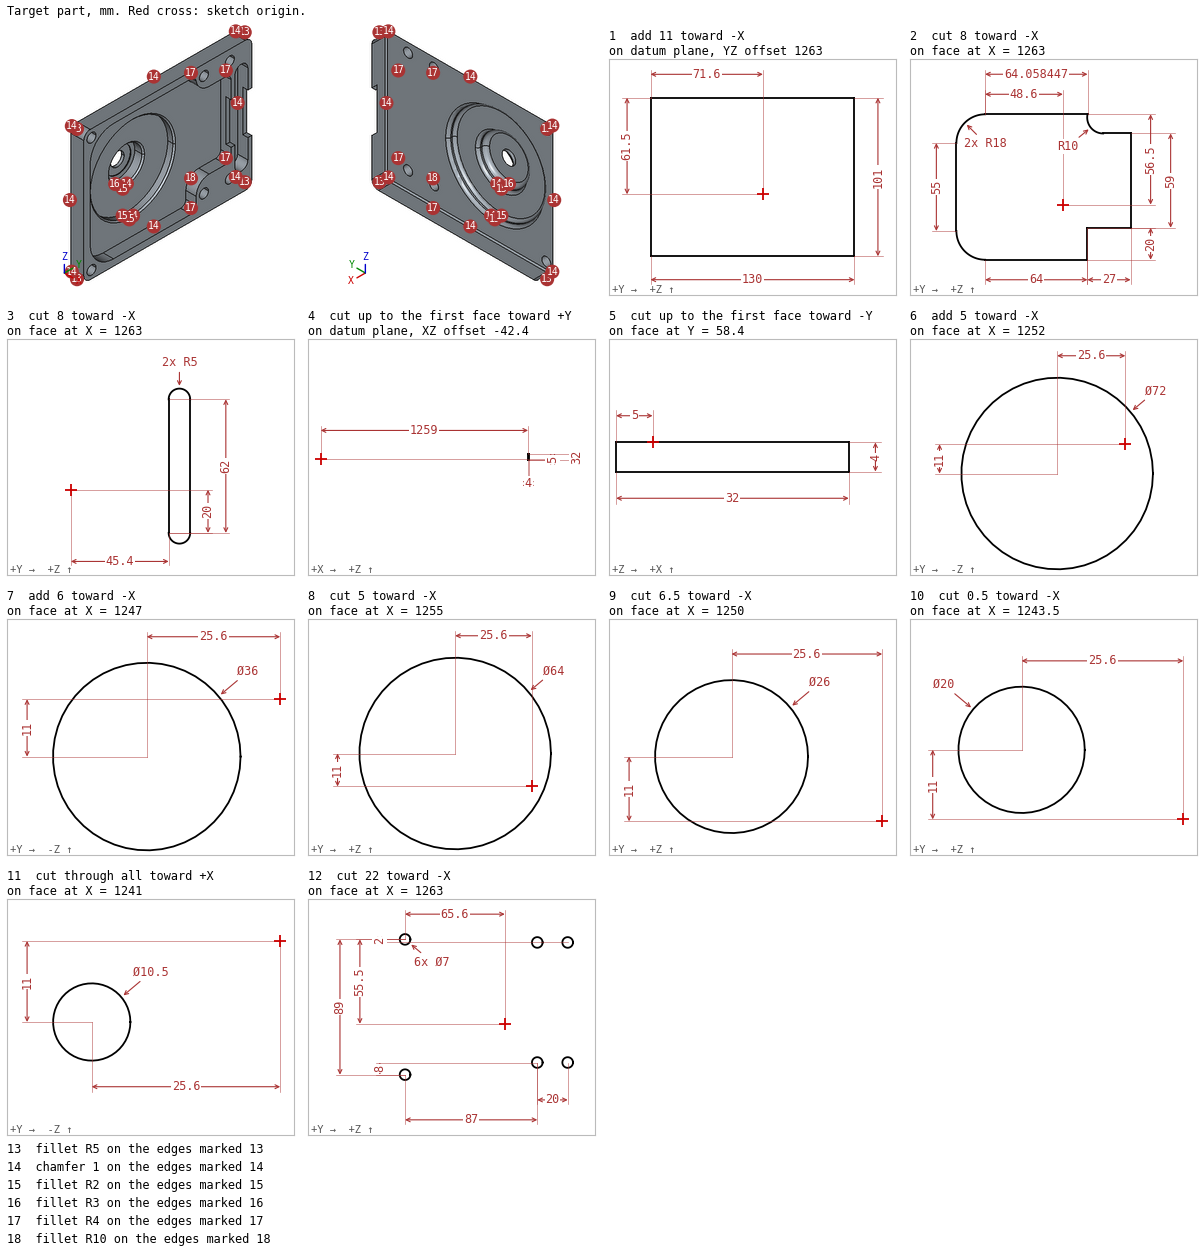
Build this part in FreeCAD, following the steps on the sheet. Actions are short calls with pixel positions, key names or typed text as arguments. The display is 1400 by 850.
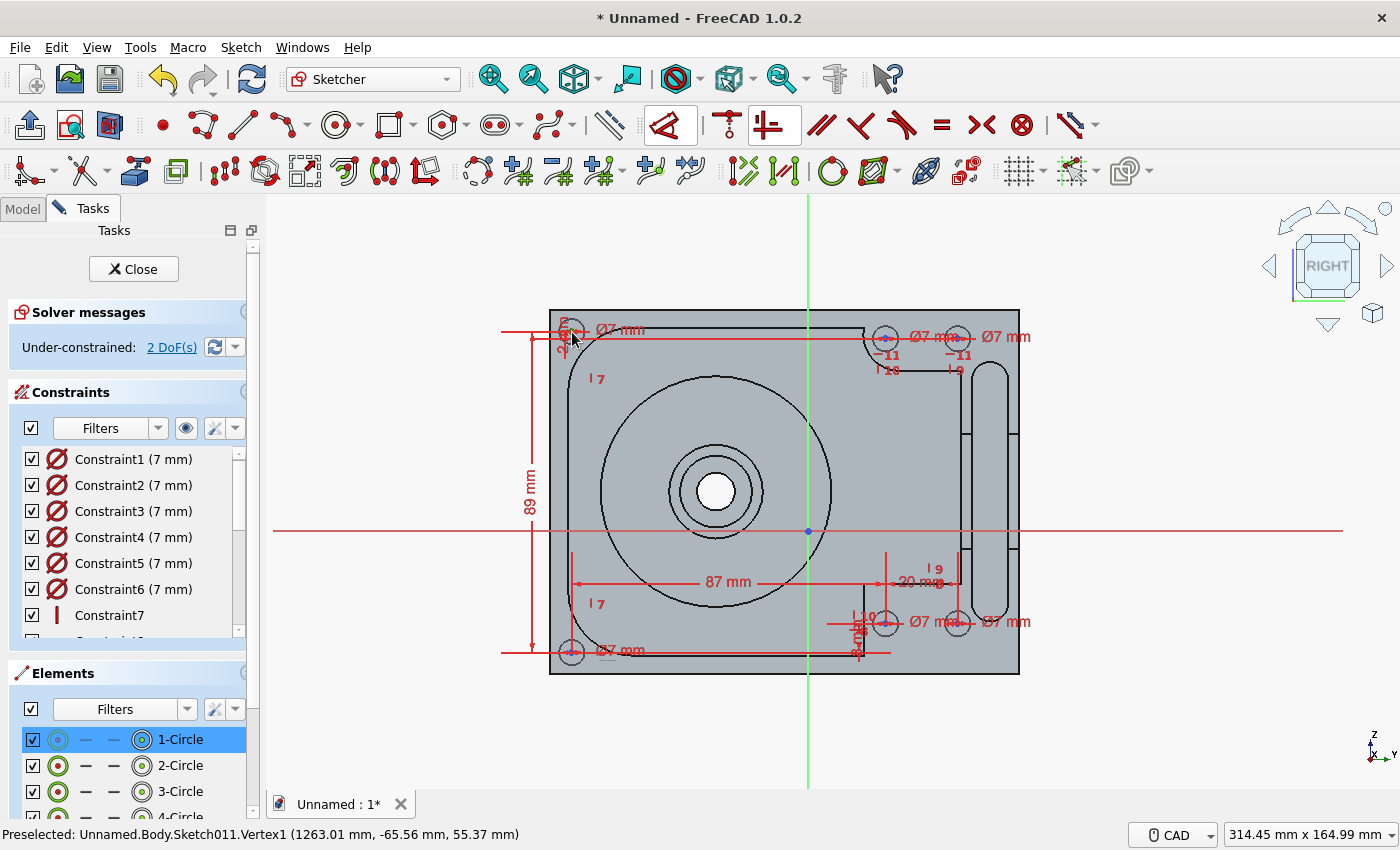
click(692, 126)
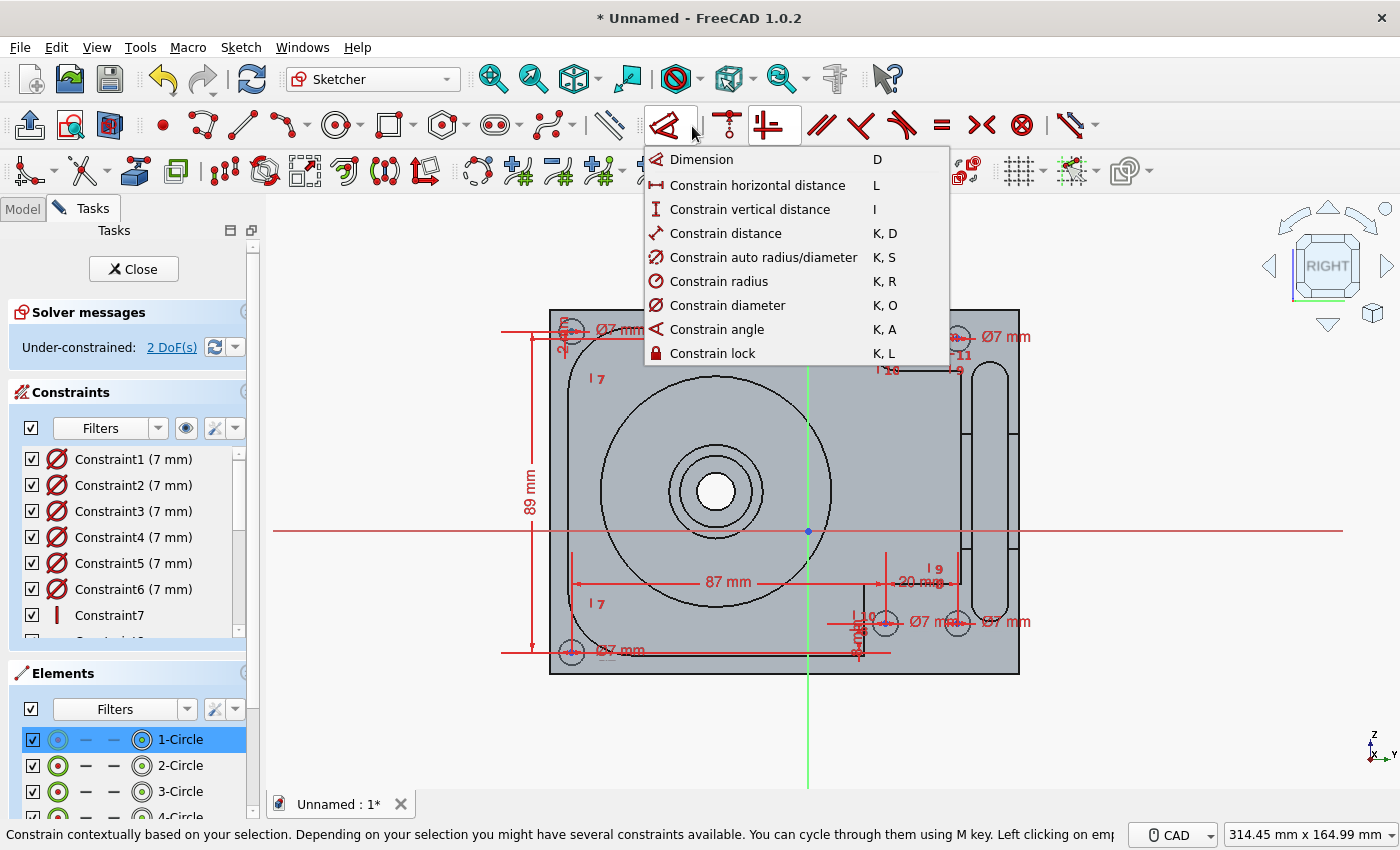
click(797, 185)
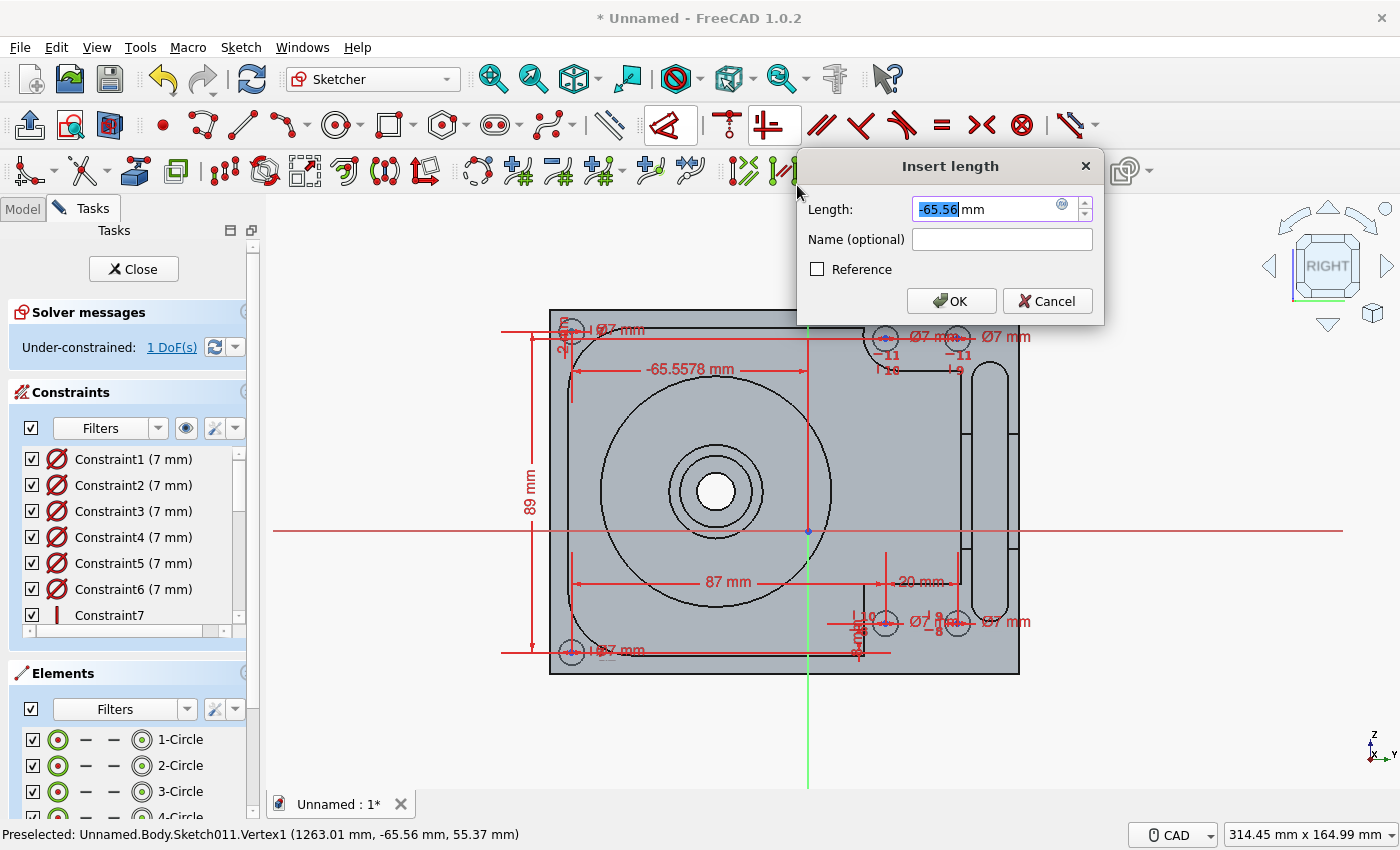
text(-65.6)
key(Return)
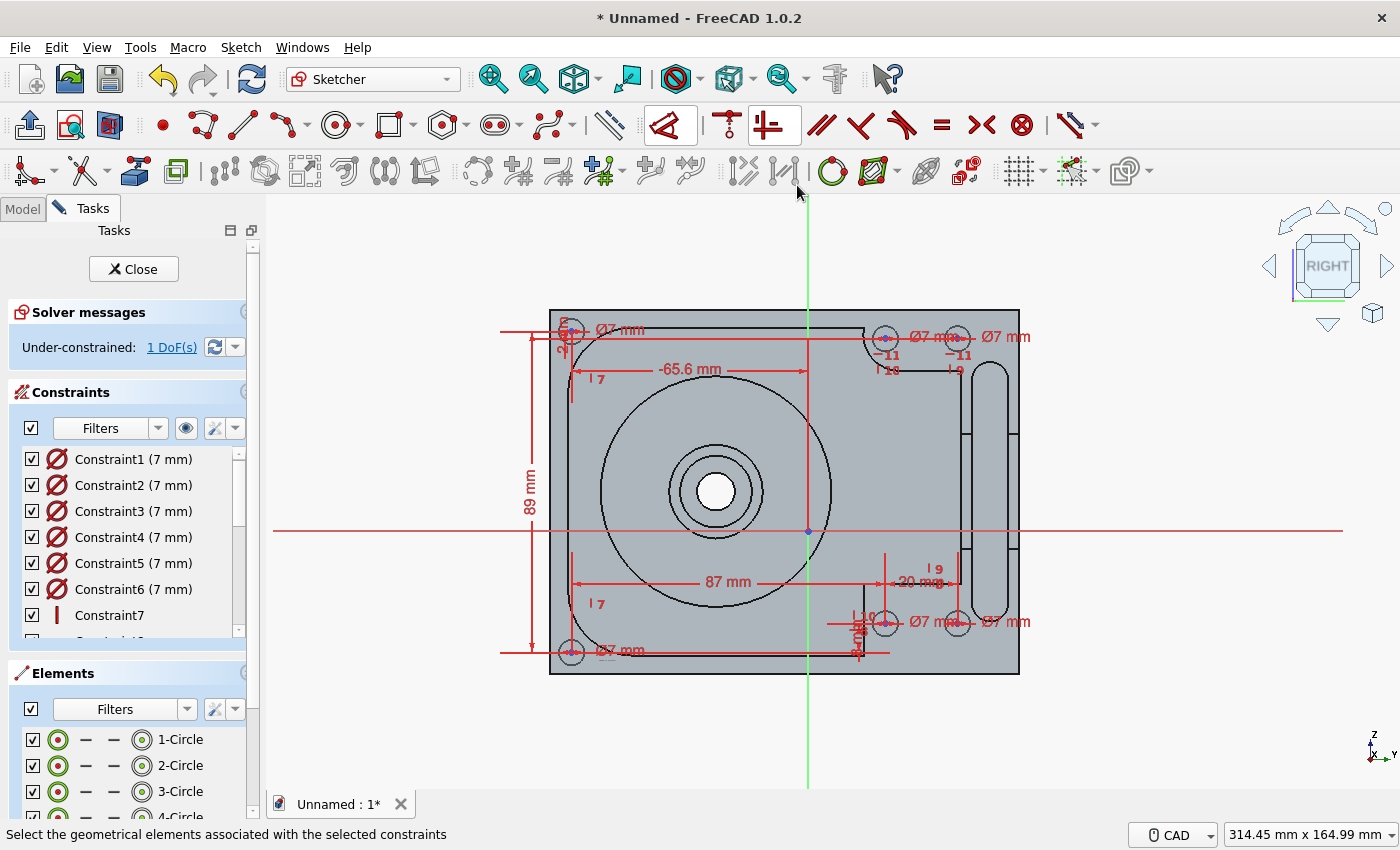
click(572, 332)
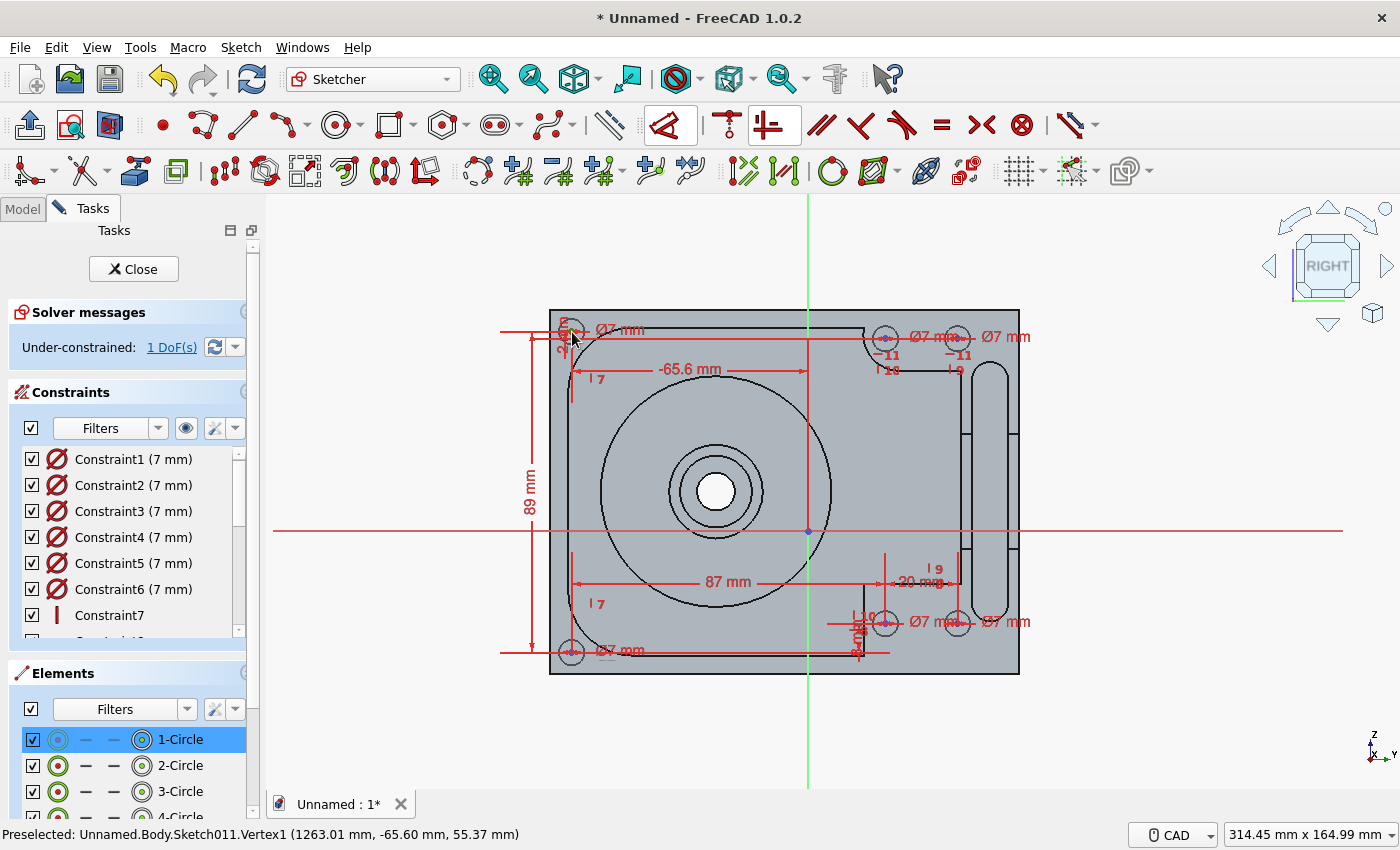
key(i)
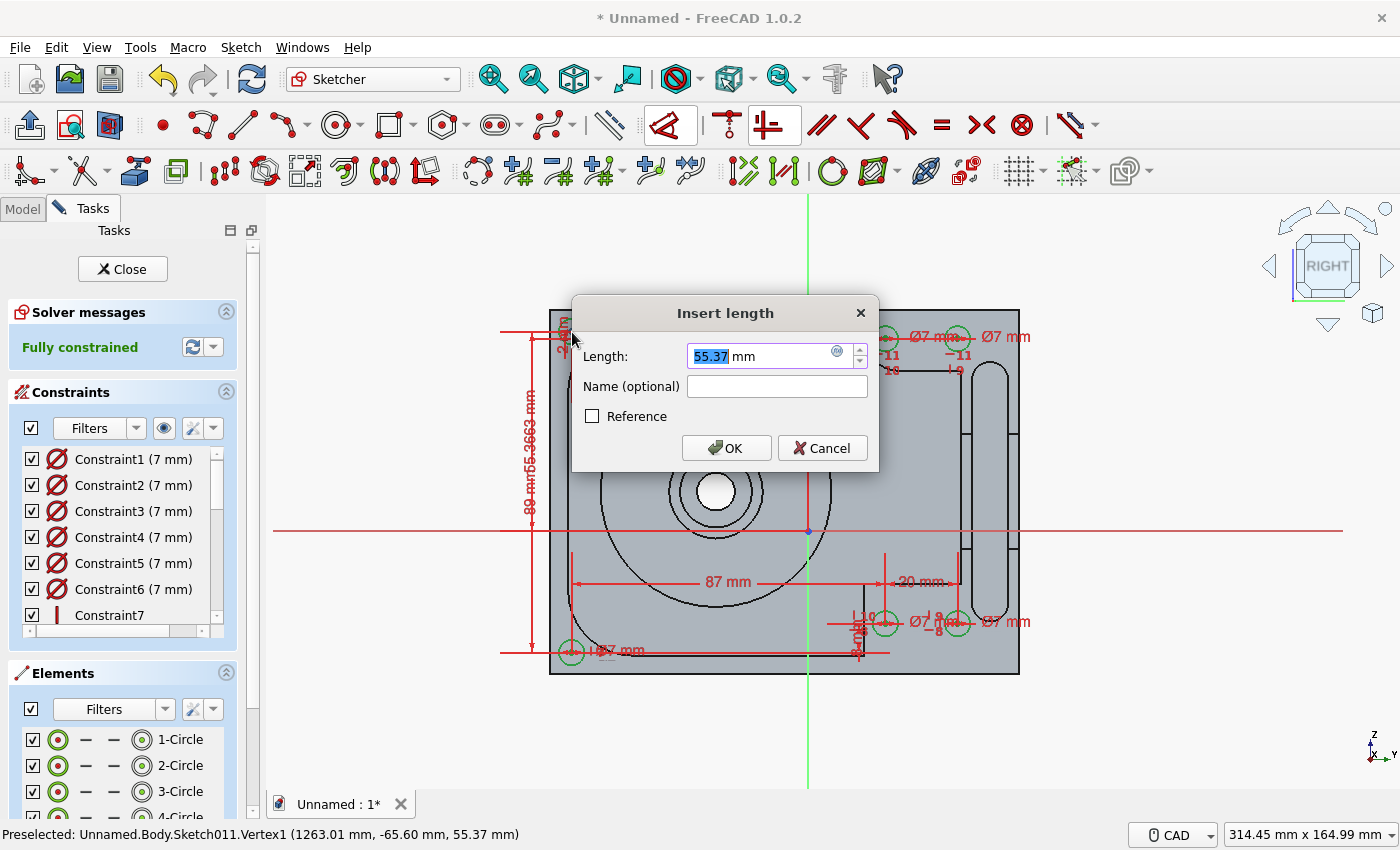
text(55.5)
key(Return)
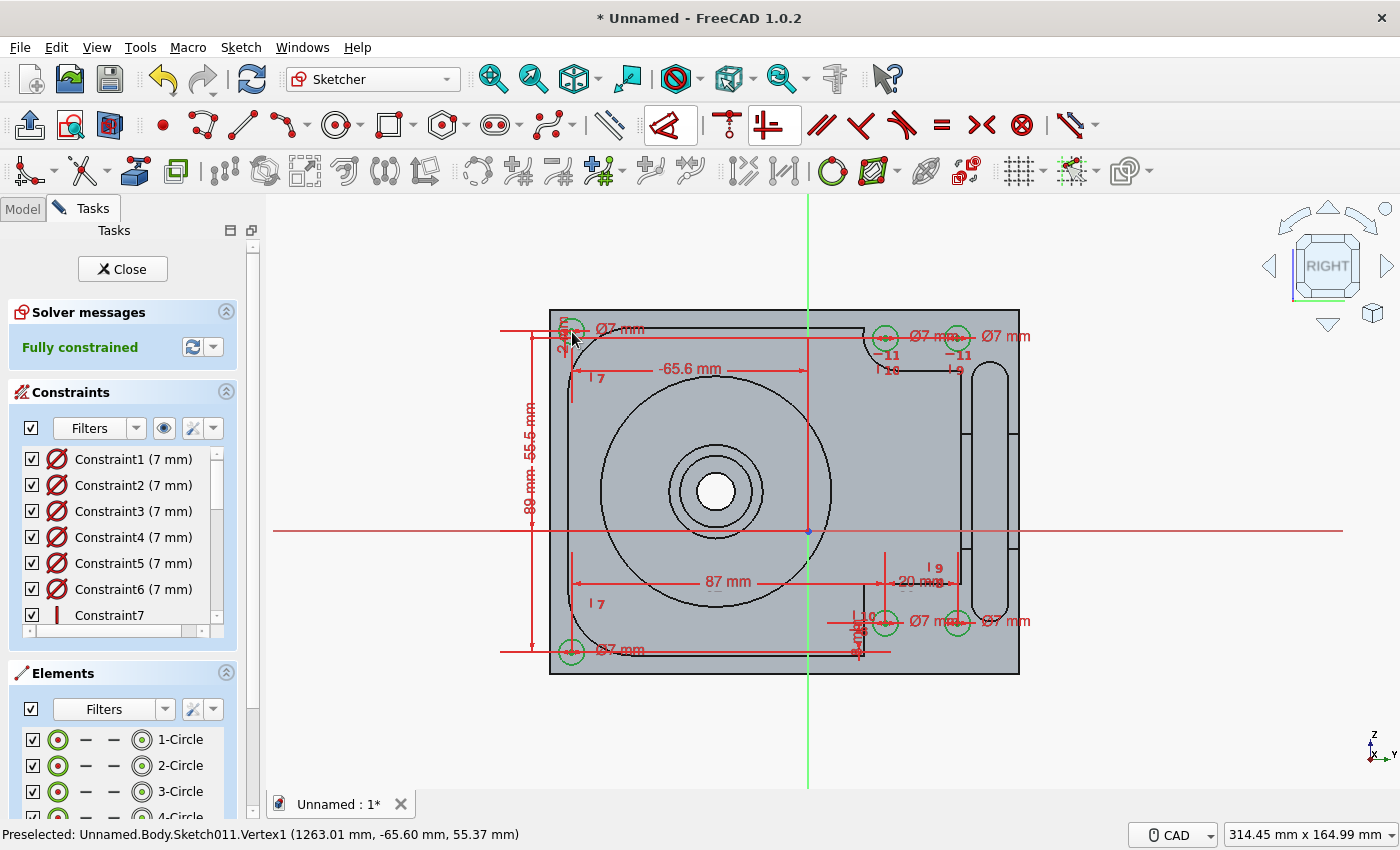
click(123, 269)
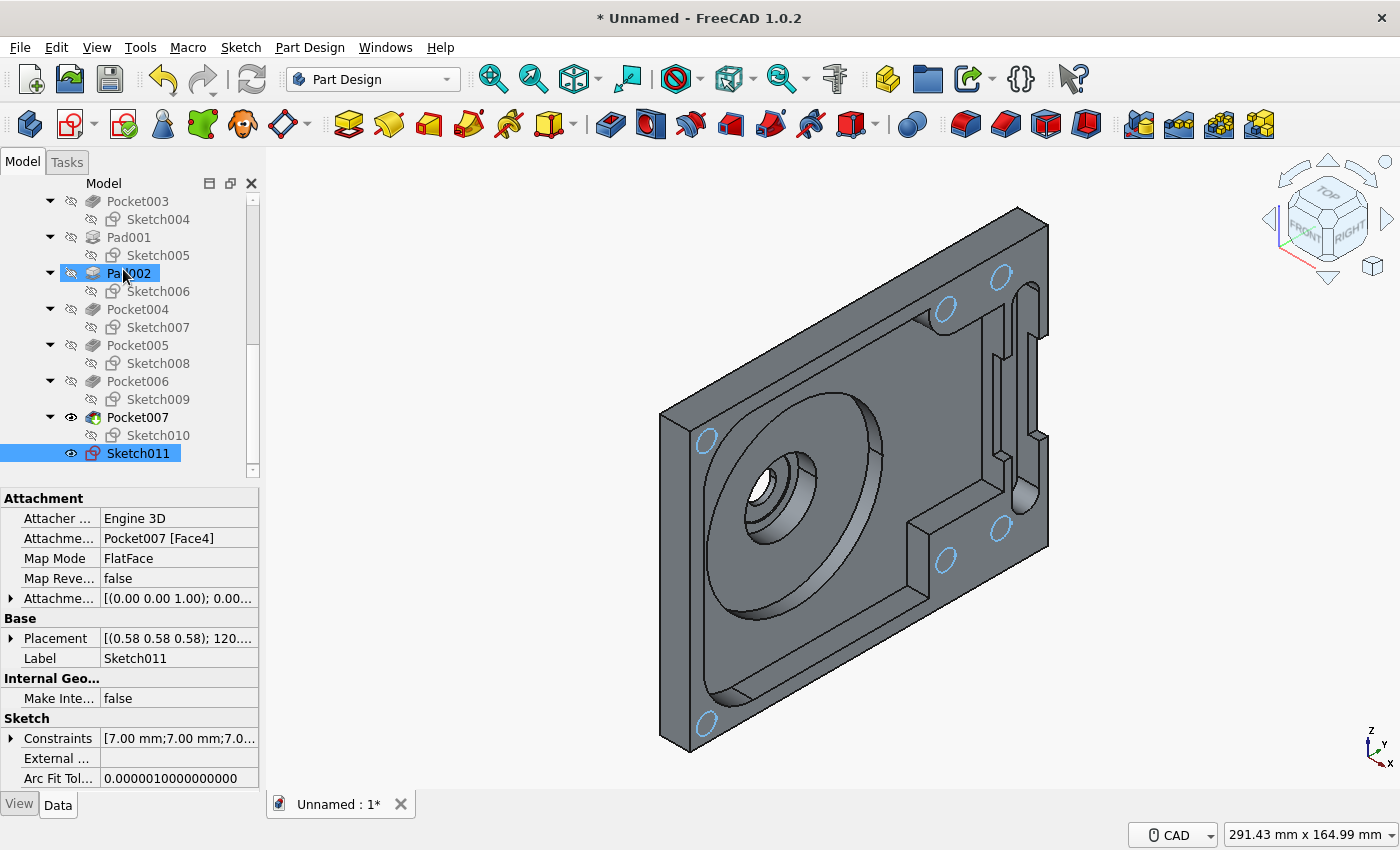
click(612, 124)